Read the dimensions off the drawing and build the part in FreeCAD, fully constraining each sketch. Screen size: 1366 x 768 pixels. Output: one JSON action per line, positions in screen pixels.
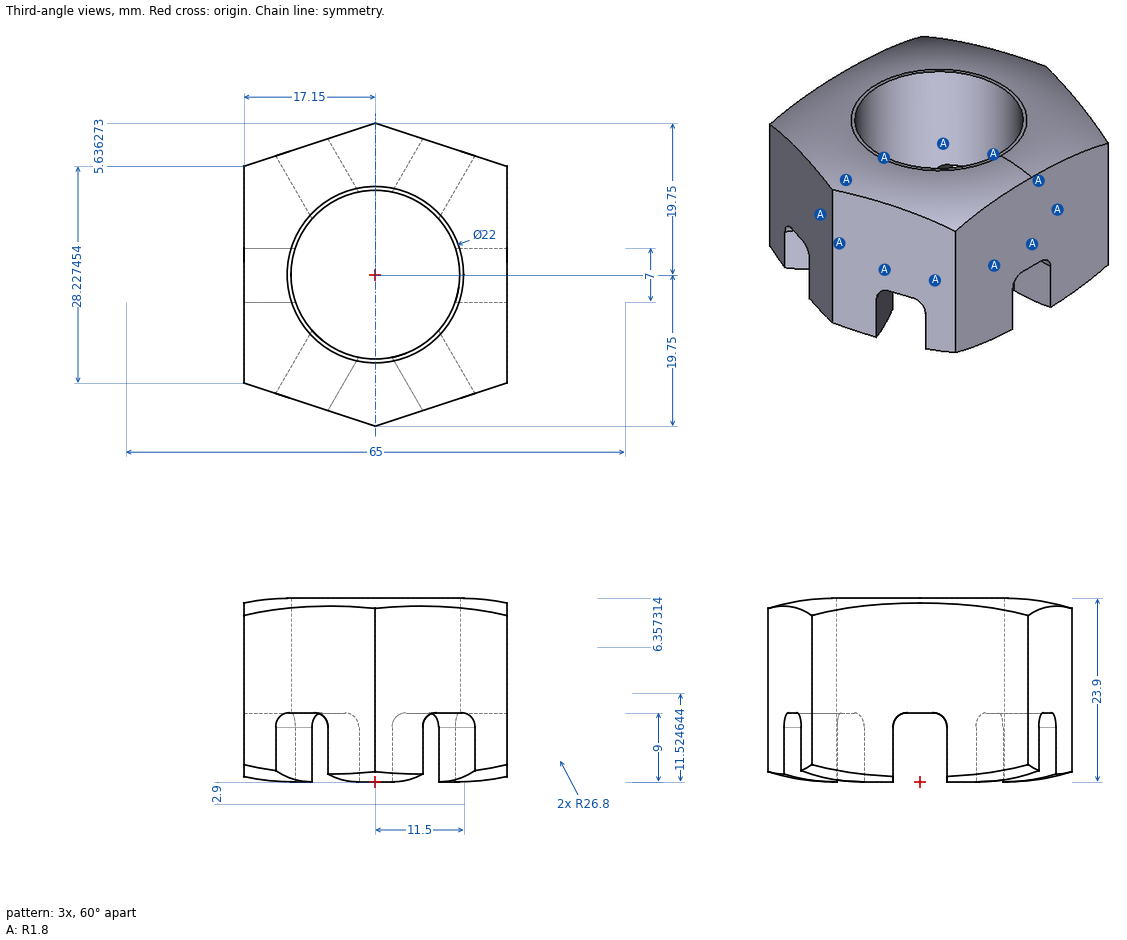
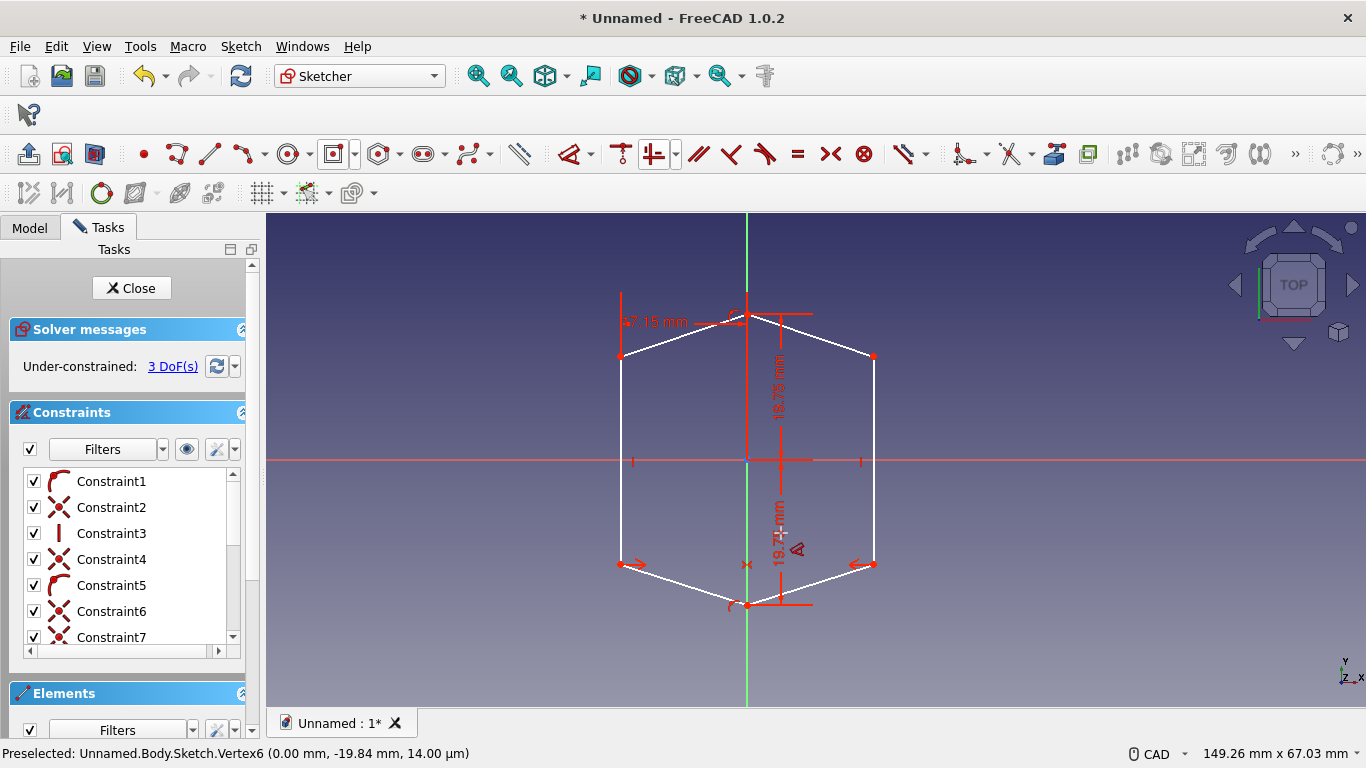
{"action": "left_click", "coordinate": [621, 419]}
{"action": "left_click", "coordinate": [587, 413]}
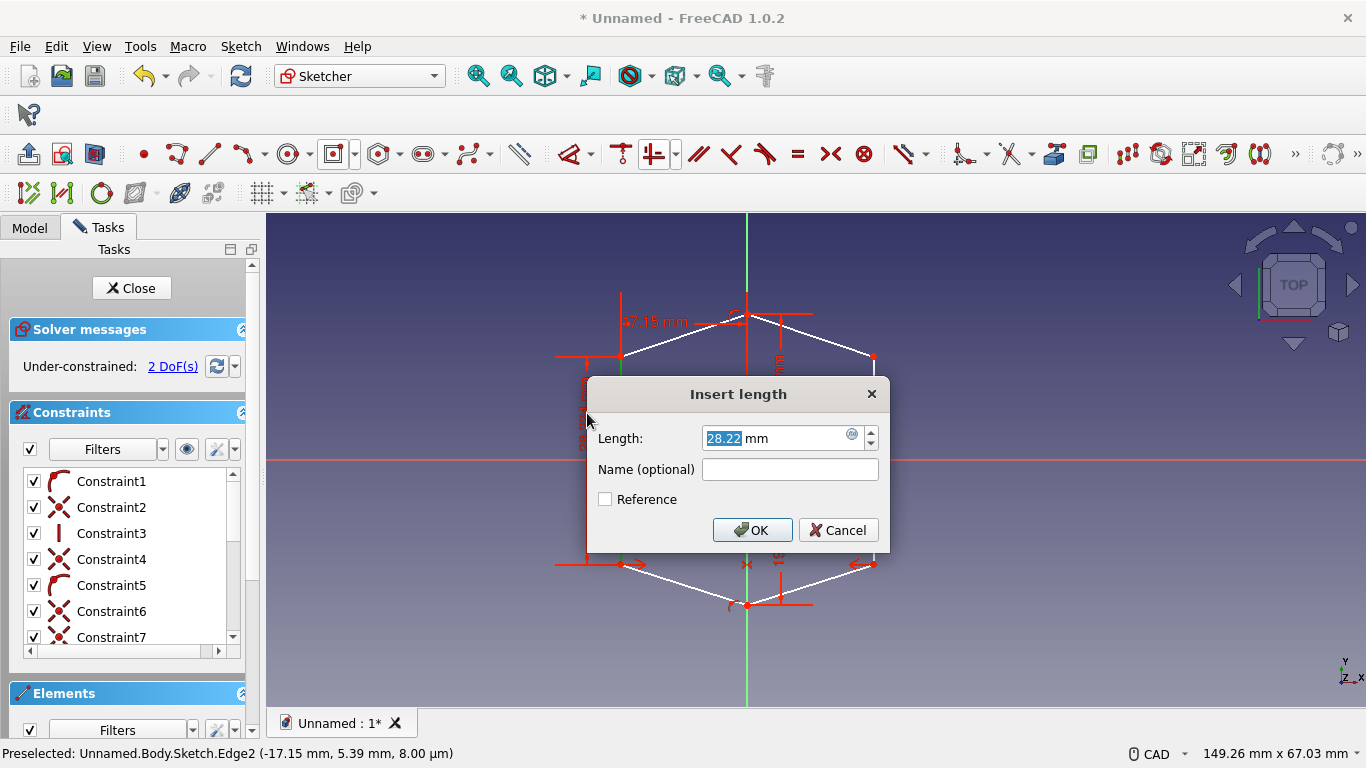
{"action": "type", "text": "28.227454"}
{"action": "key", "text": "Return"}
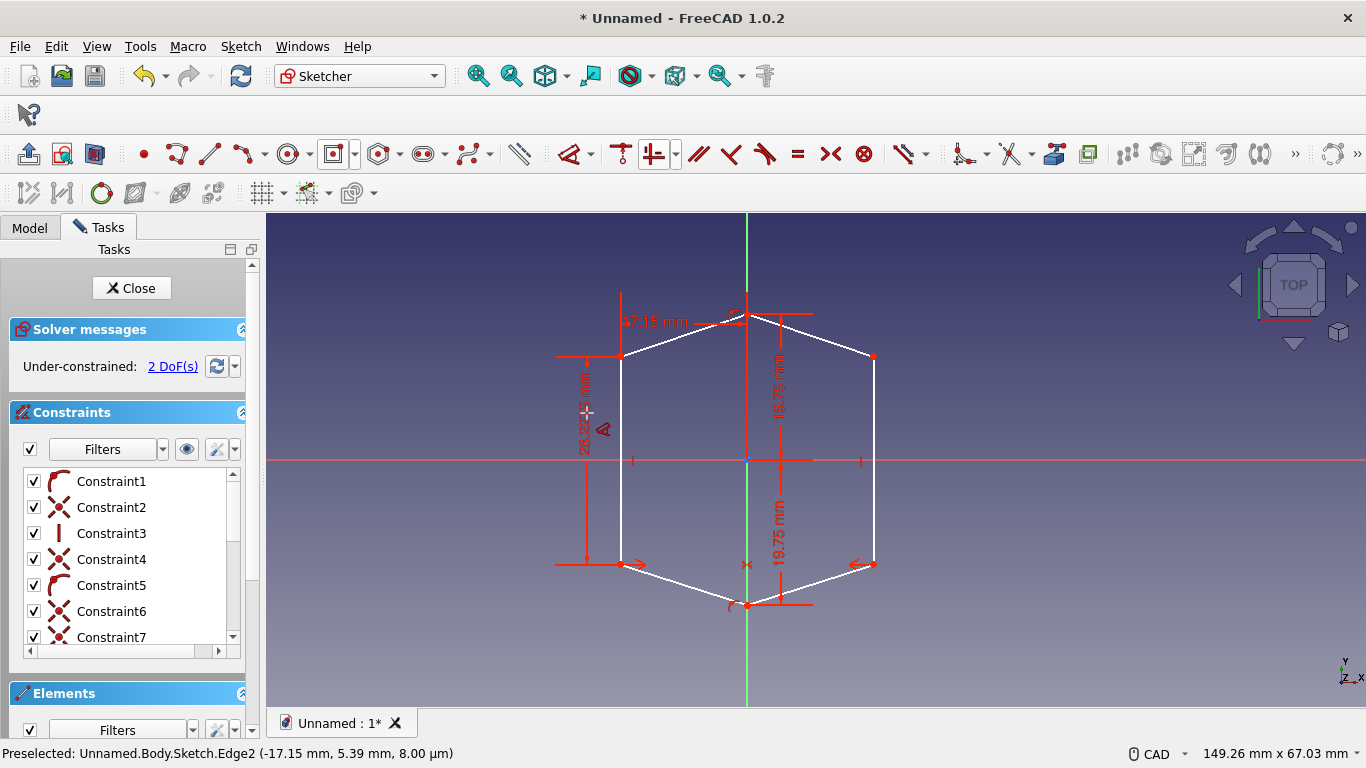
{"action": "left_click", "coordinate": [874, 503]}
{"action": "left_click", "coordinate": [908, 413]}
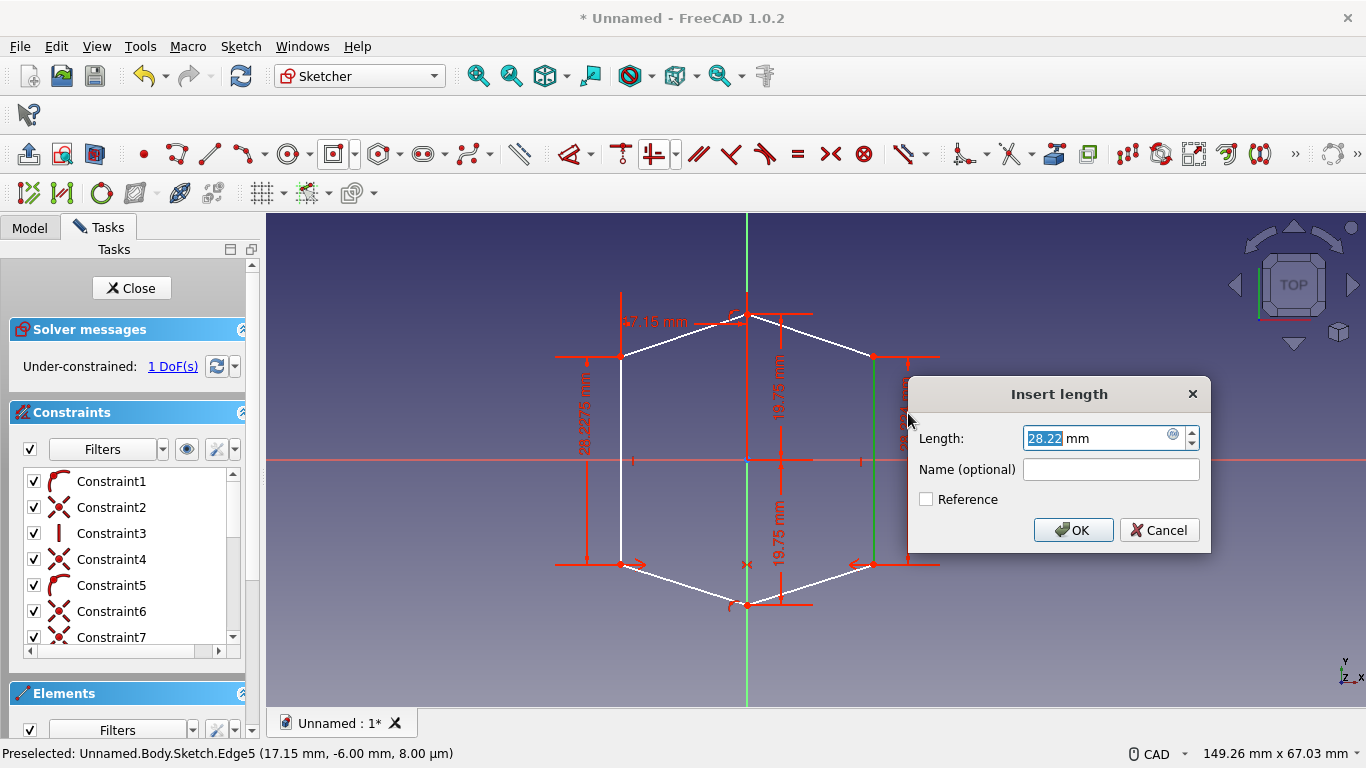
{"action": "type", "text": "28.227454"}
{"action": "key", "text": "Return"}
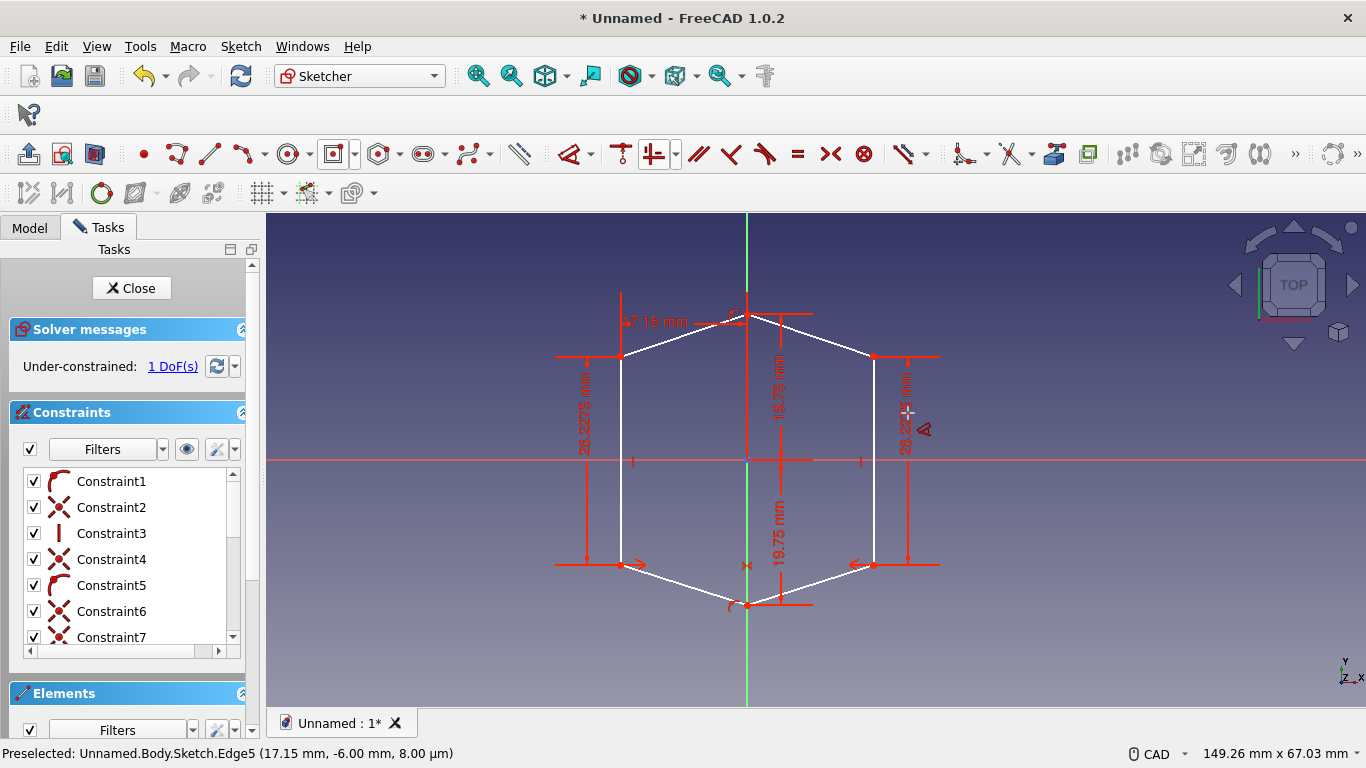
{"action": "left_click", "coordinate": [709, 327]}
{"action": "left_click", "coordinate": [587, 345]}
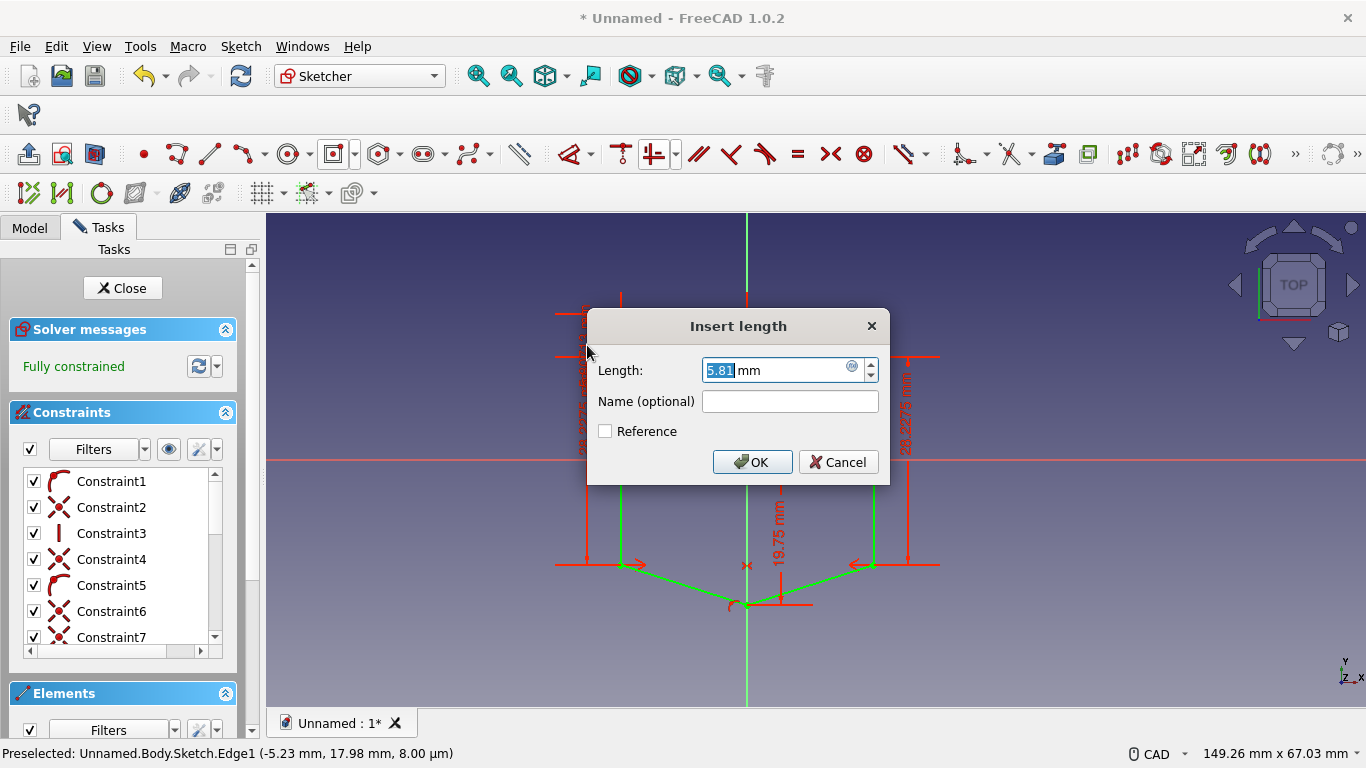
{"action": "type", "text": "5.636273"}
{"action": "key", "text": "Return"}
{"action": "key", "text": "Escape"}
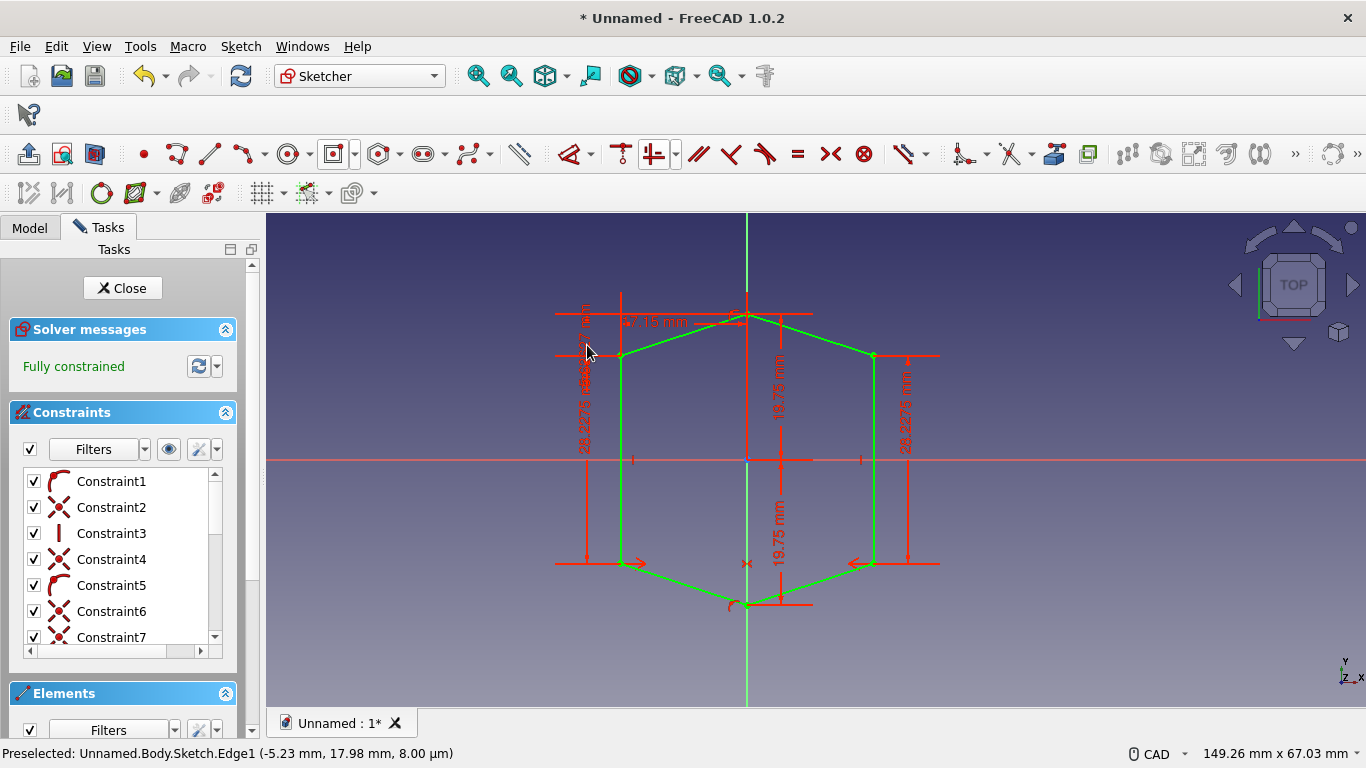
{"action": "left_click", "coordinate": [123, 288]}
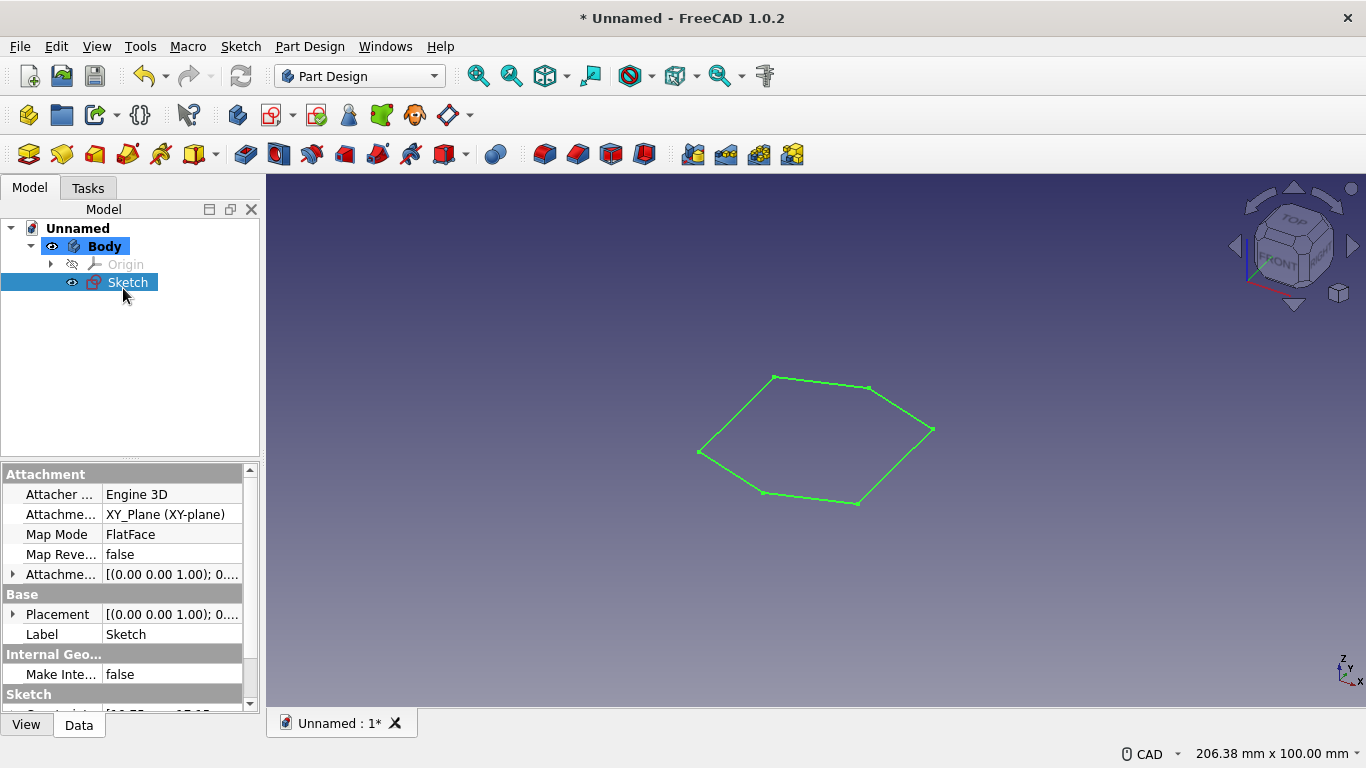
{"action": "left_click", "coordinate": [29, 154]}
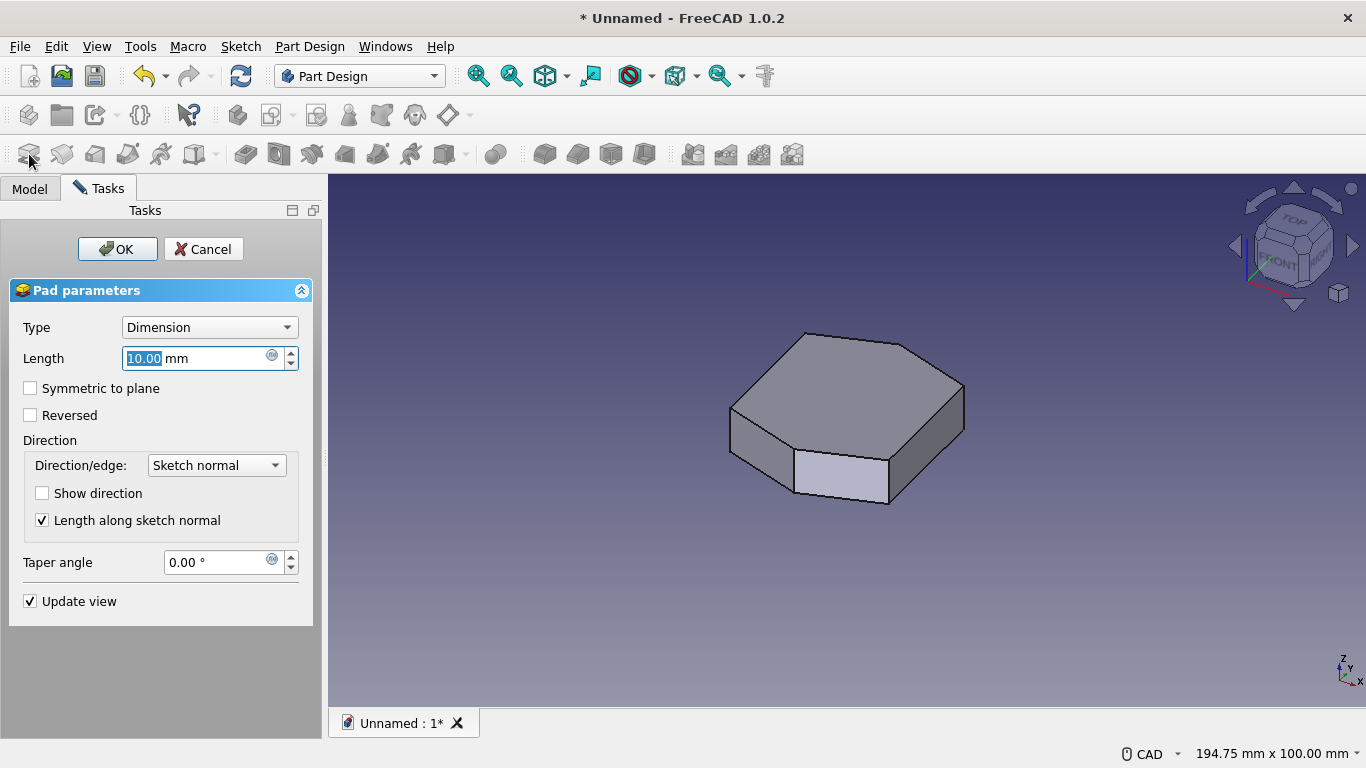
{"action": "type", "text": "23.9"}
{"action": "key", "text": "Tab"}